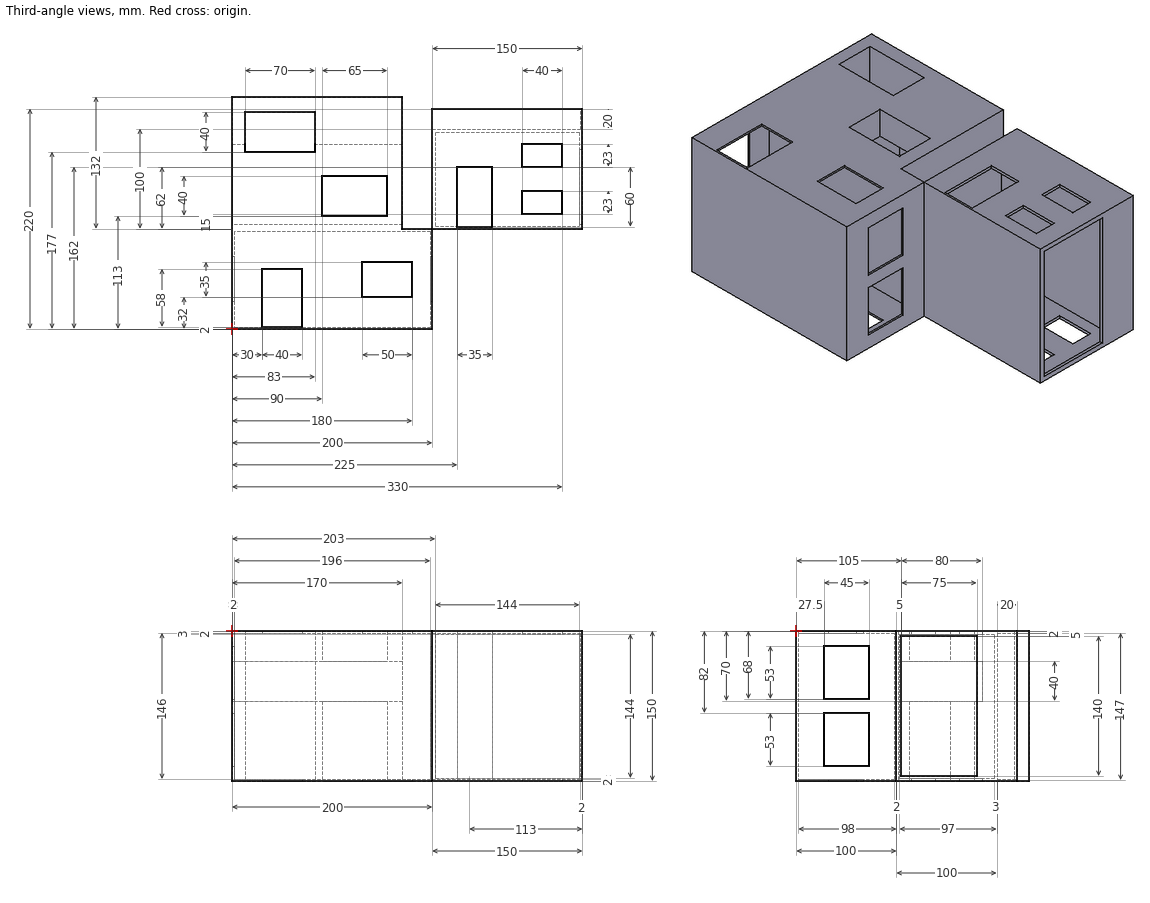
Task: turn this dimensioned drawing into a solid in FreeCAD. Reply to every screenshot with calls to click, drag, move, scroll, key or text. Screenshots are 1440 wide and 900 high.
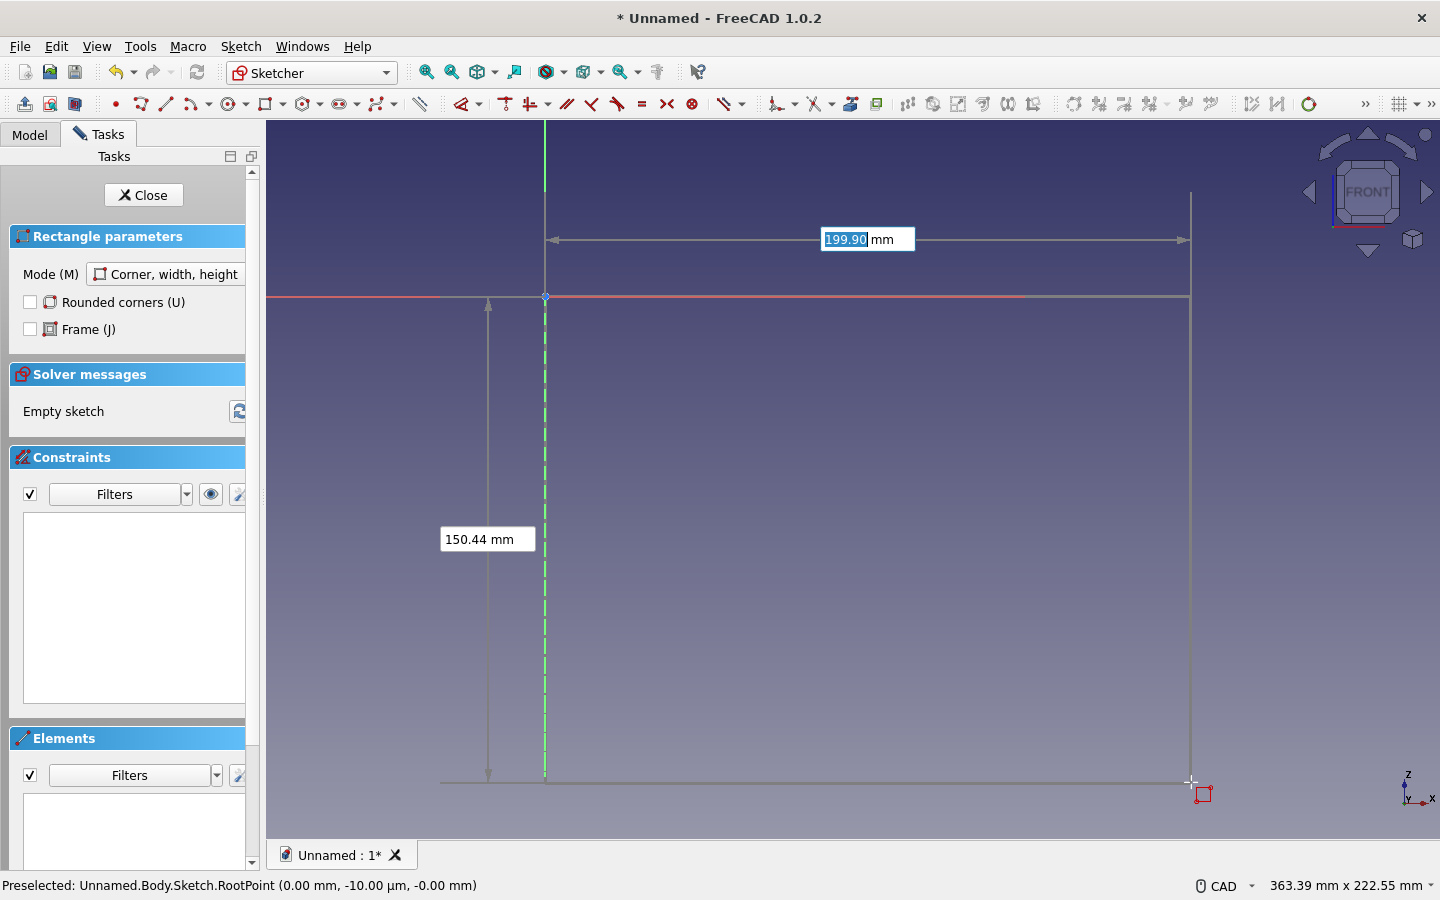
text(200)
key(Tab)
text(150)
key(Return)
key(Escape)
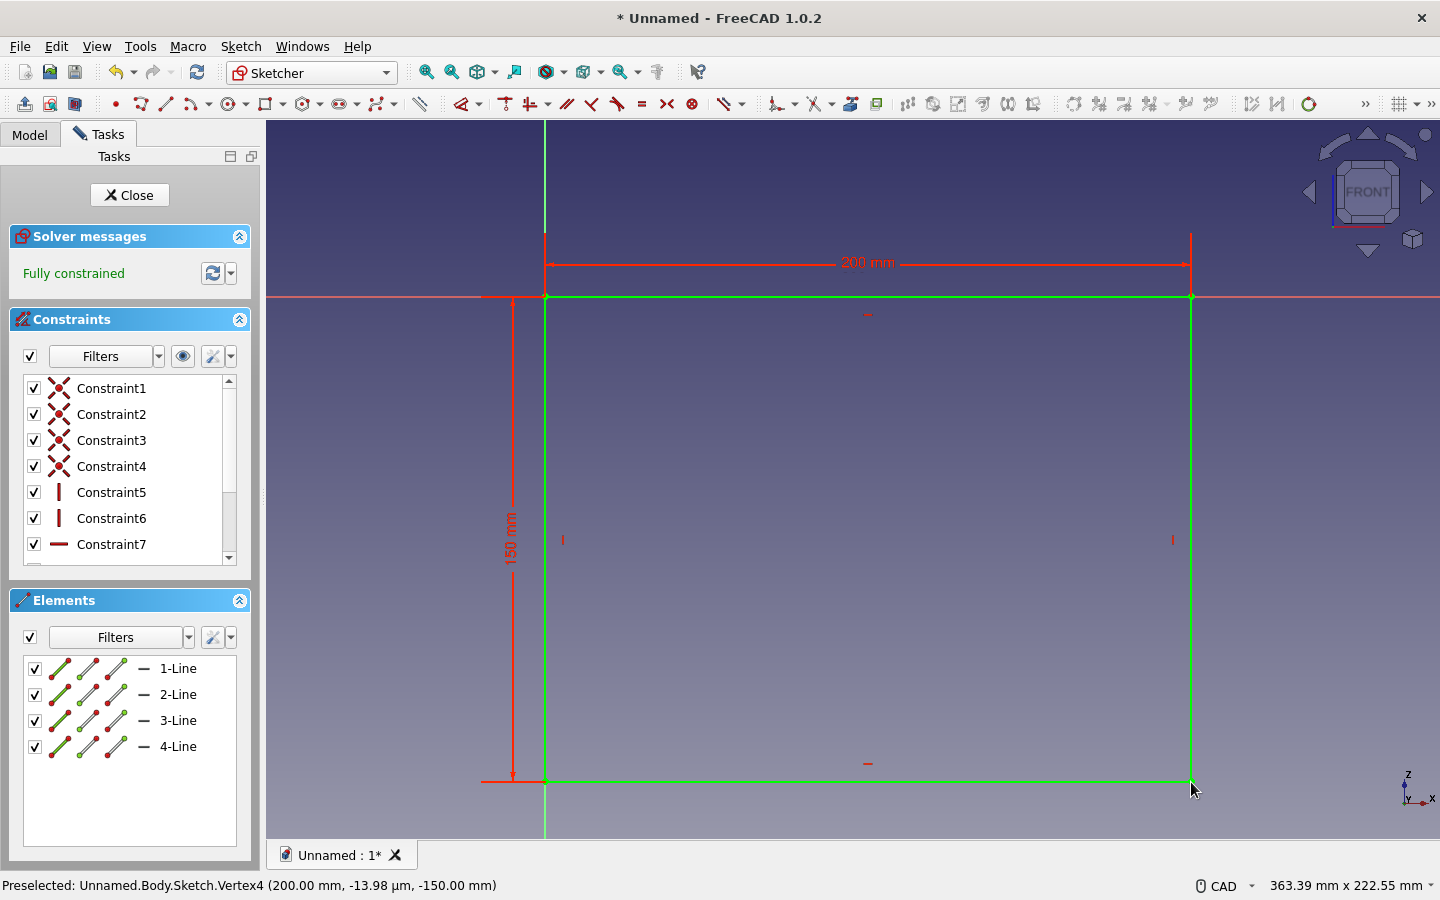
click(130, 195)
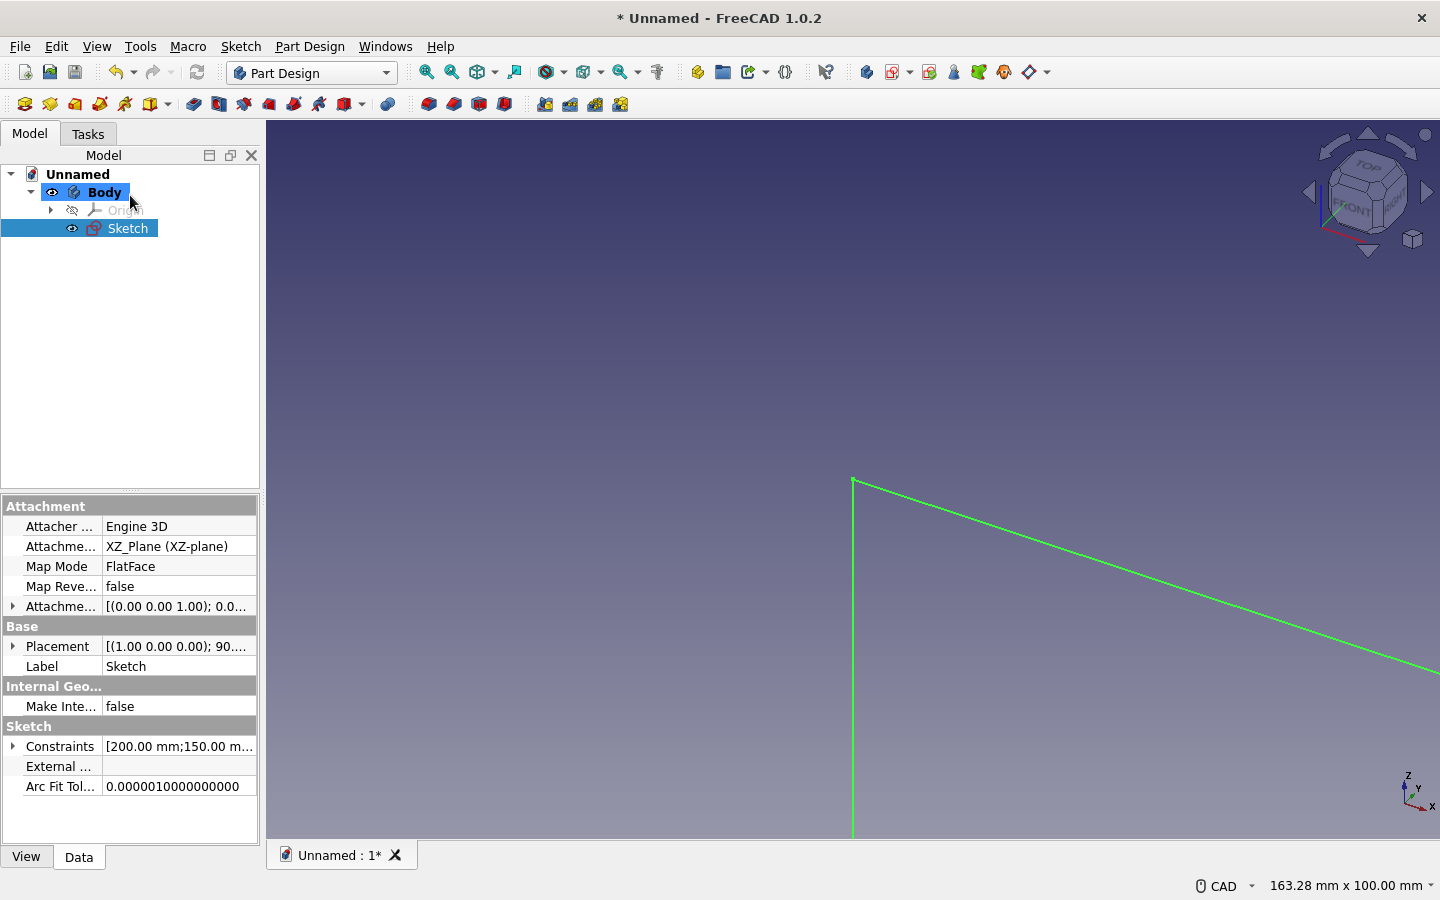
click(25, 104)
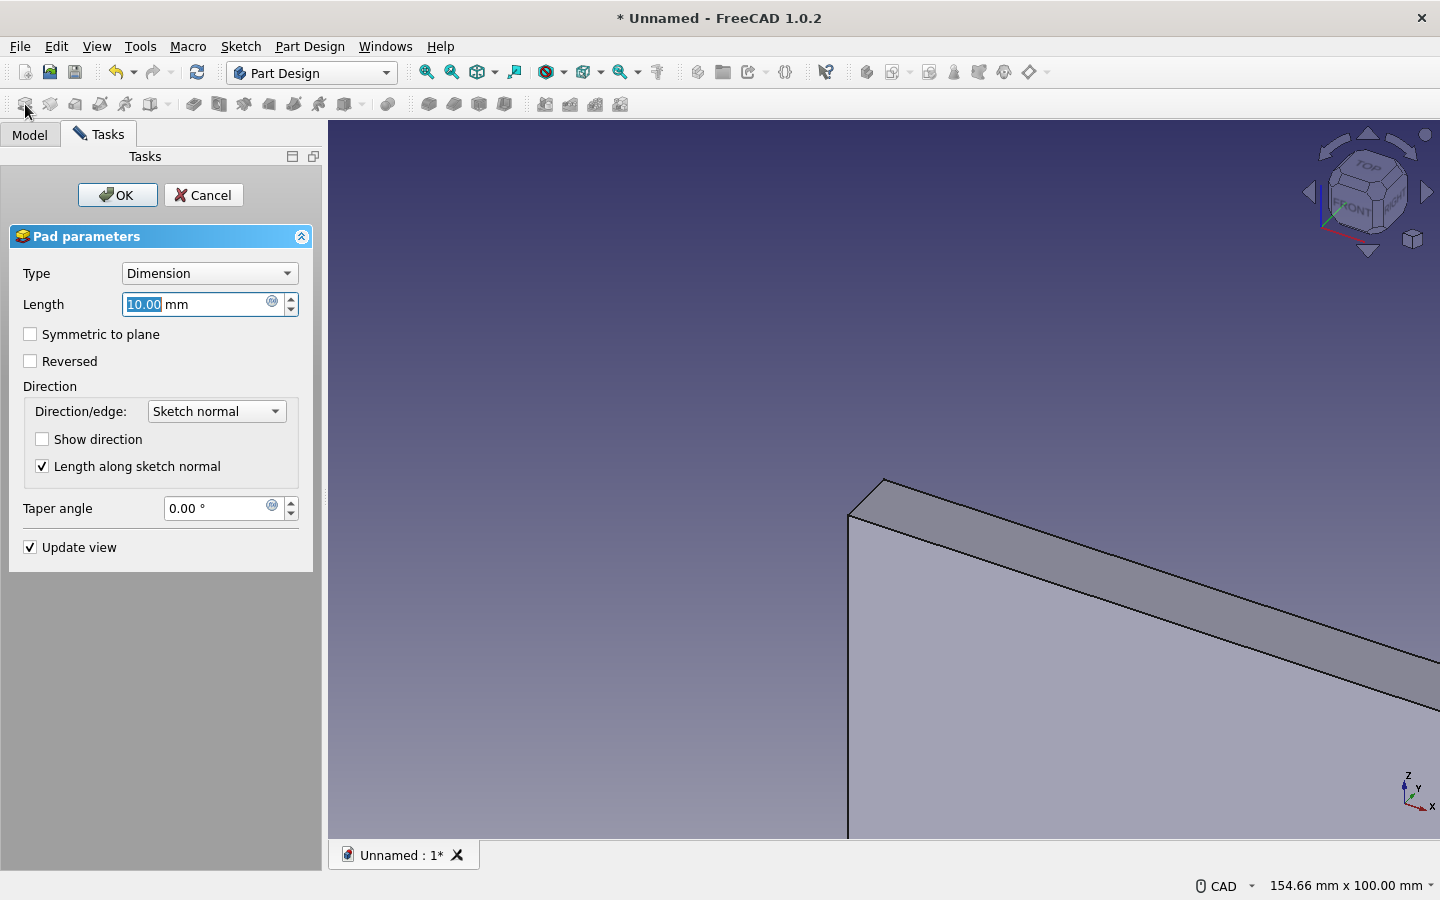
text(100)
key(Tab)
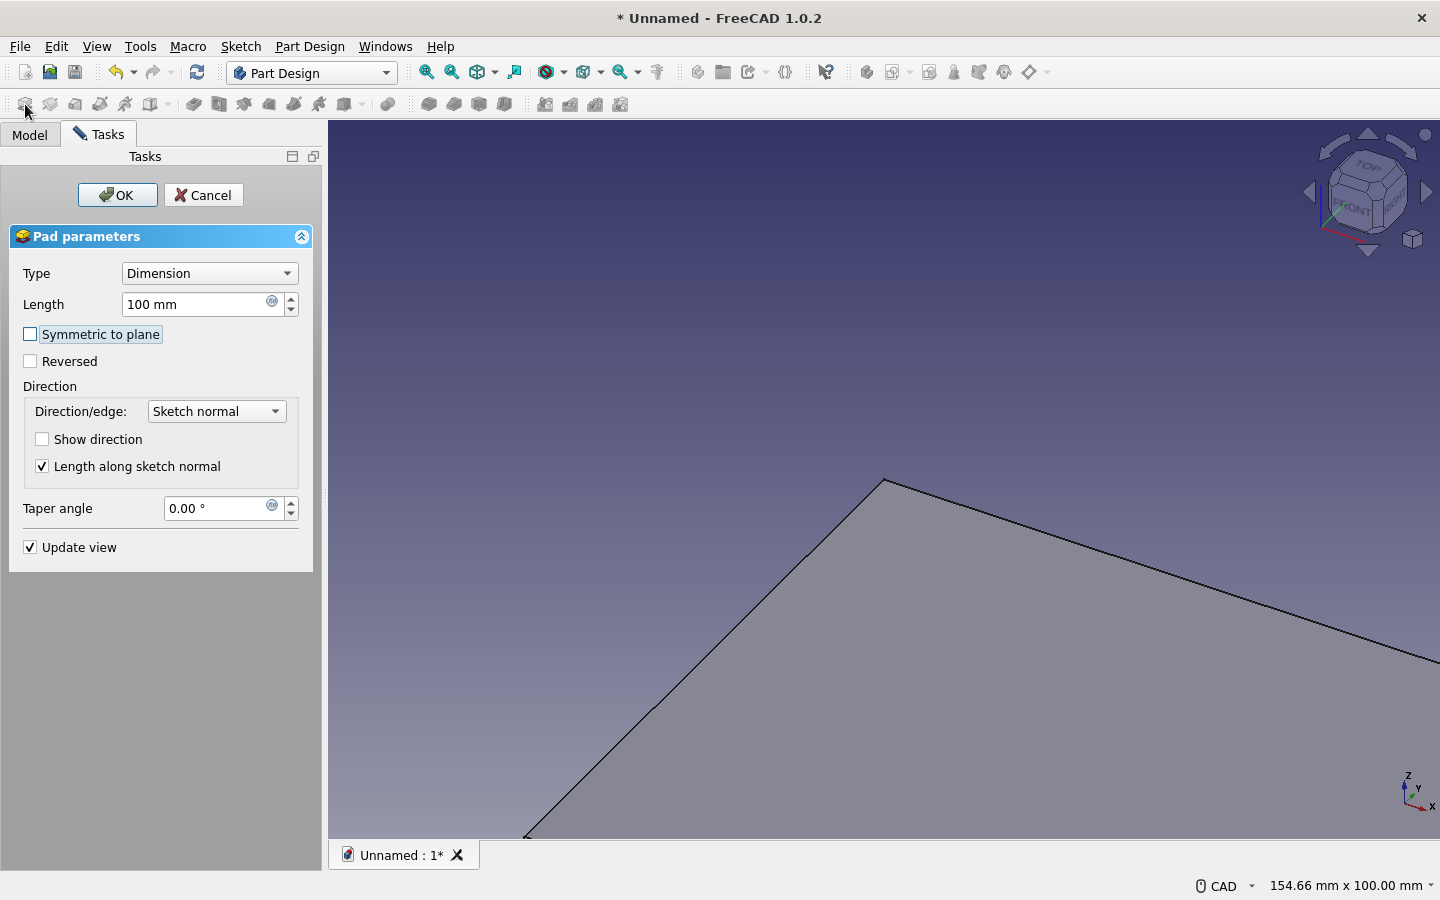
click(31, 361)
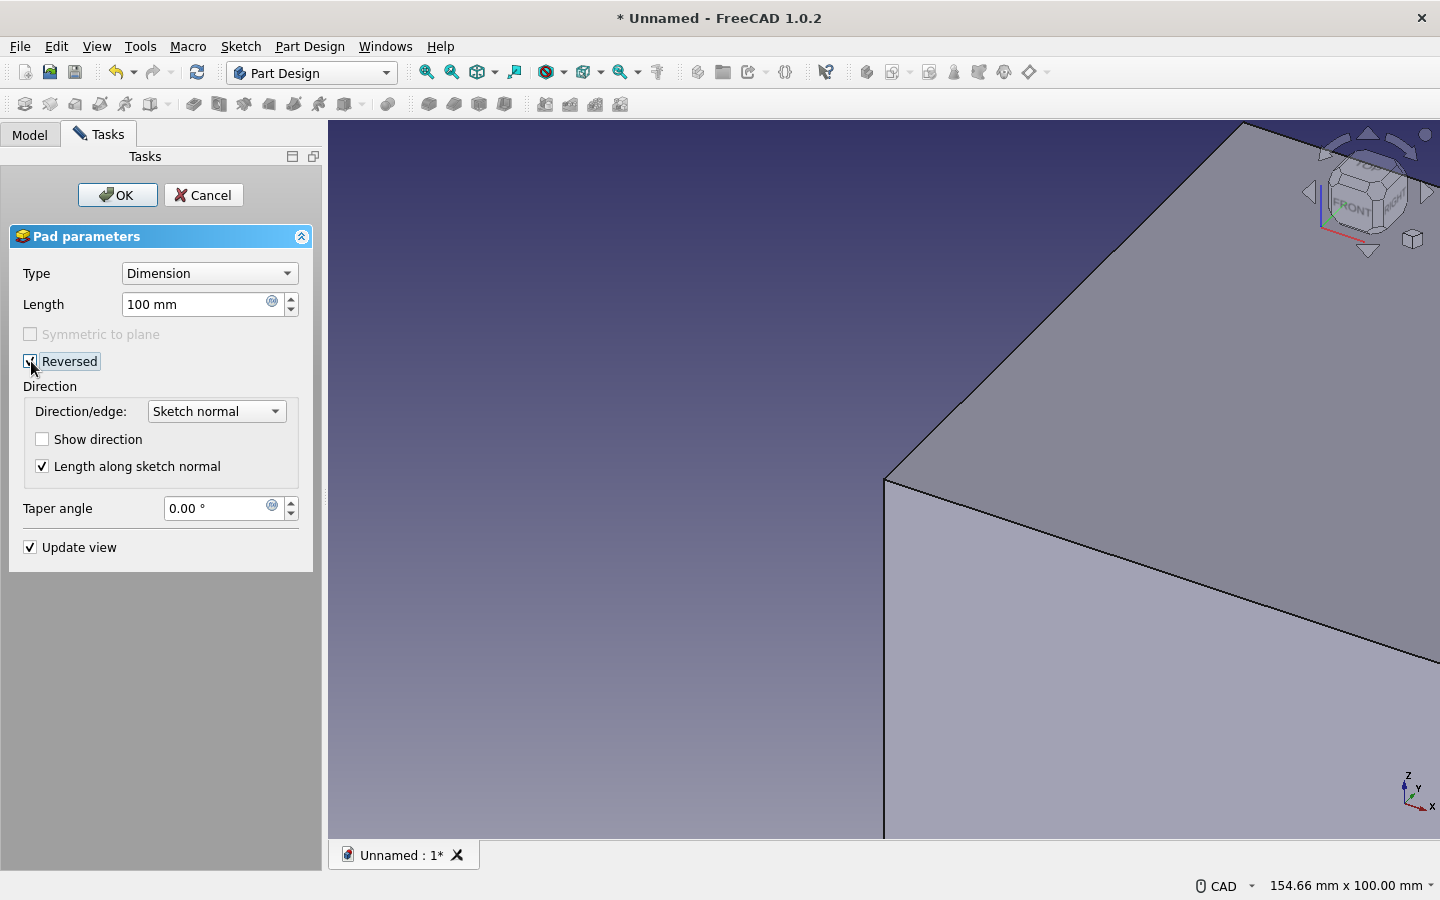
click(118, 195)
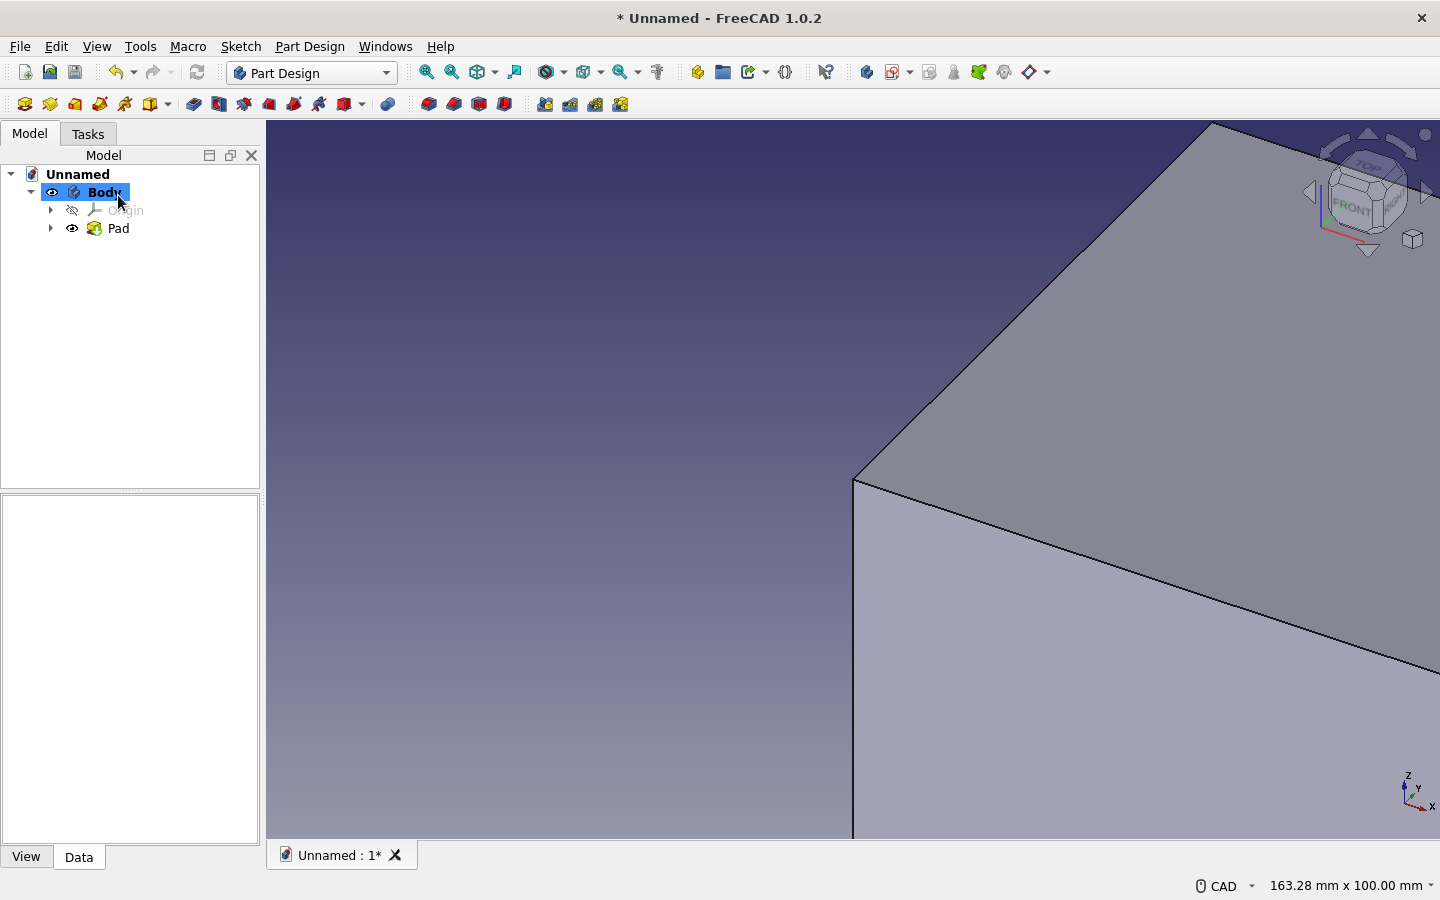
click(427, 72)